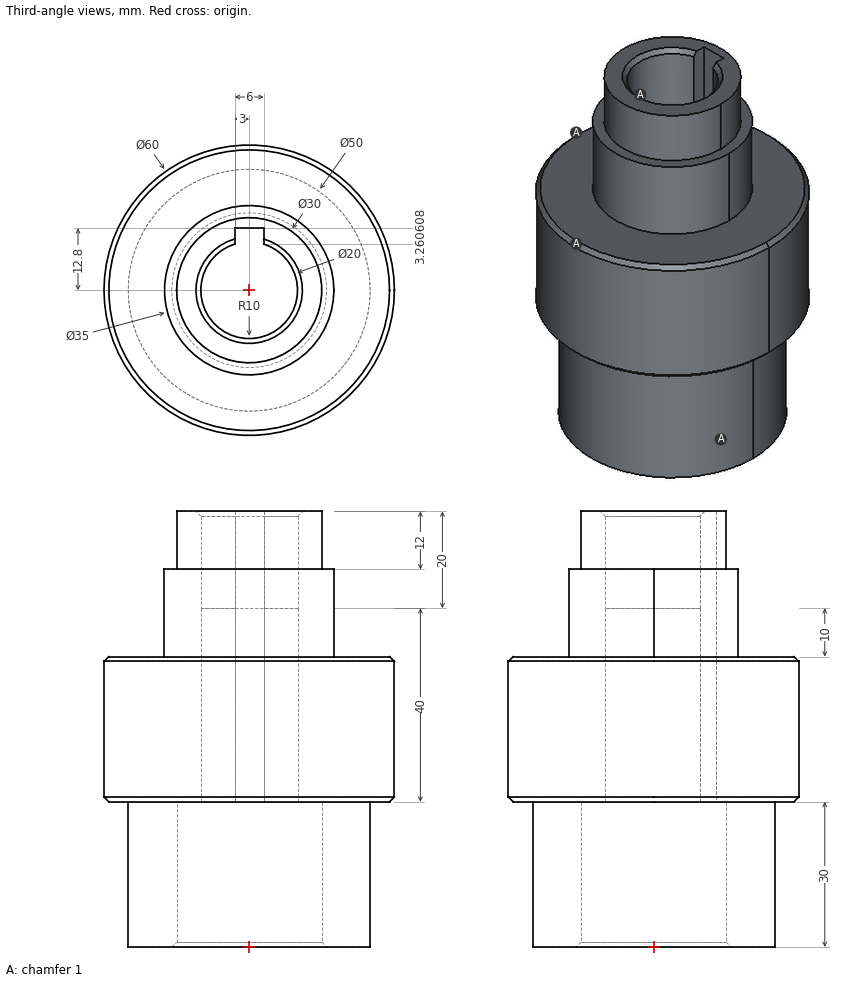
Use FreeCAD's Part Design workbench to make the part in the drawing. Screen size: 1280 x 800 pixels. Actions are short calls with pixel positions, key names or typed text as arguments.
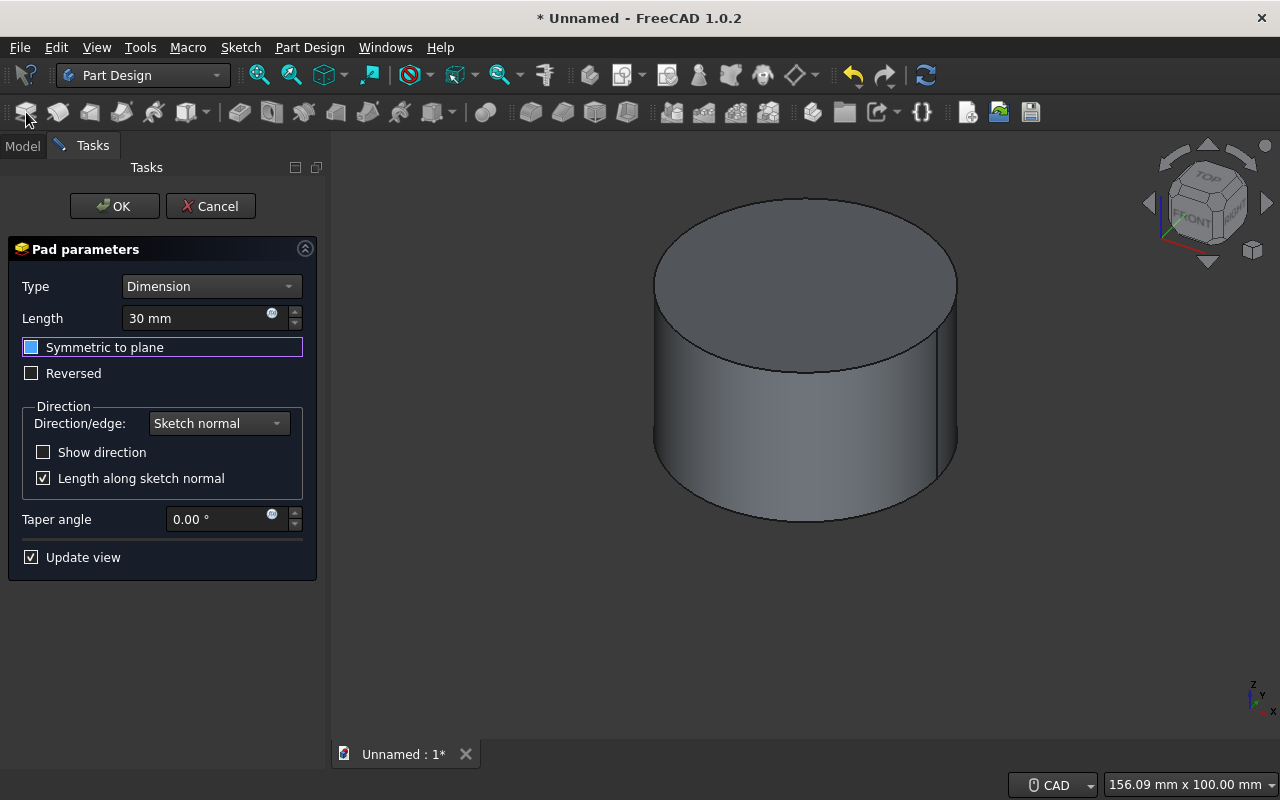
click(115, 206)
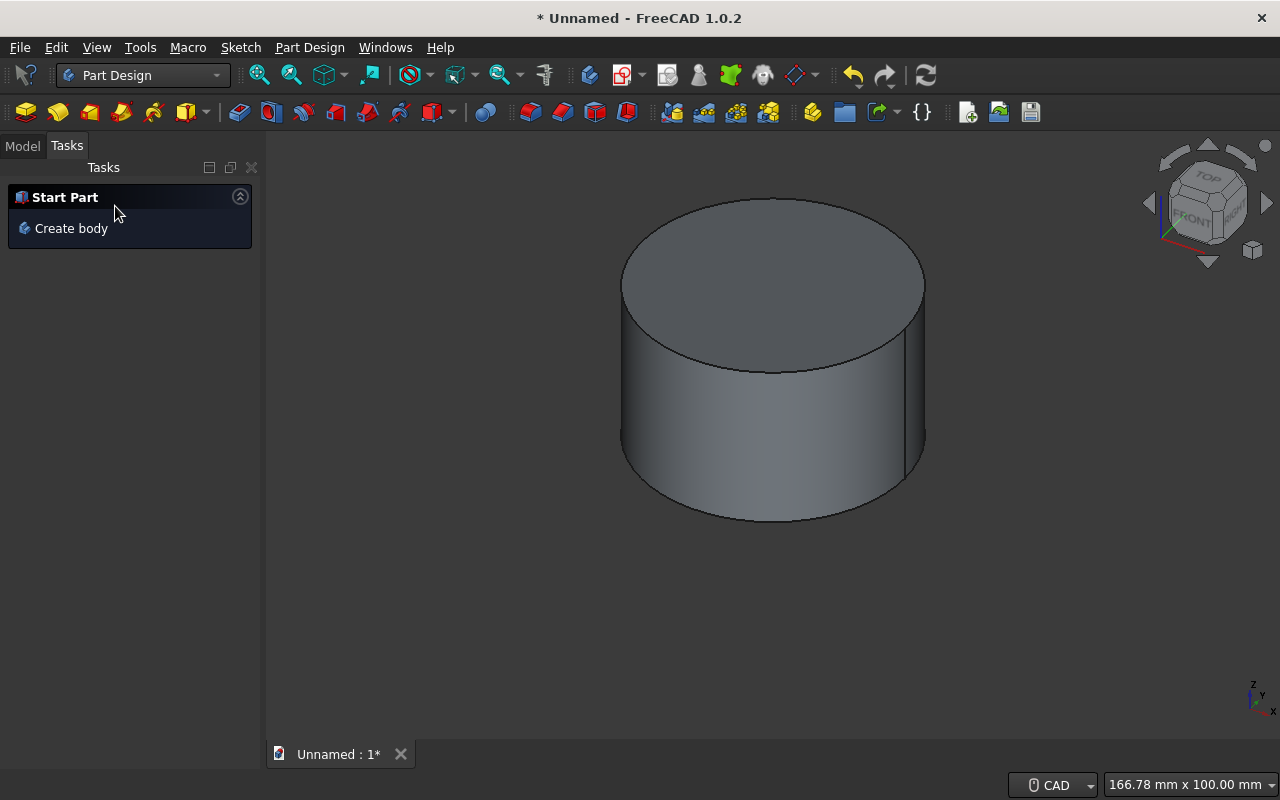
click(773, 285)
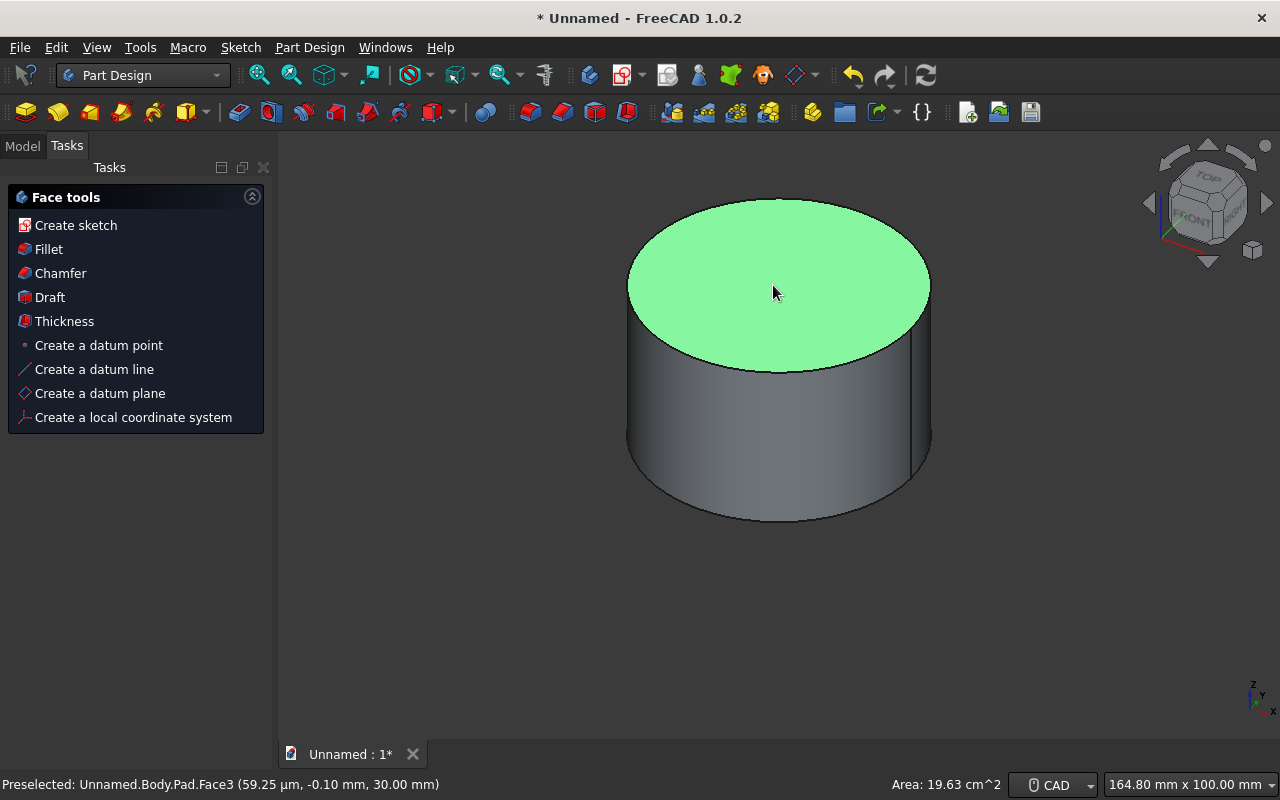
click(622, 76)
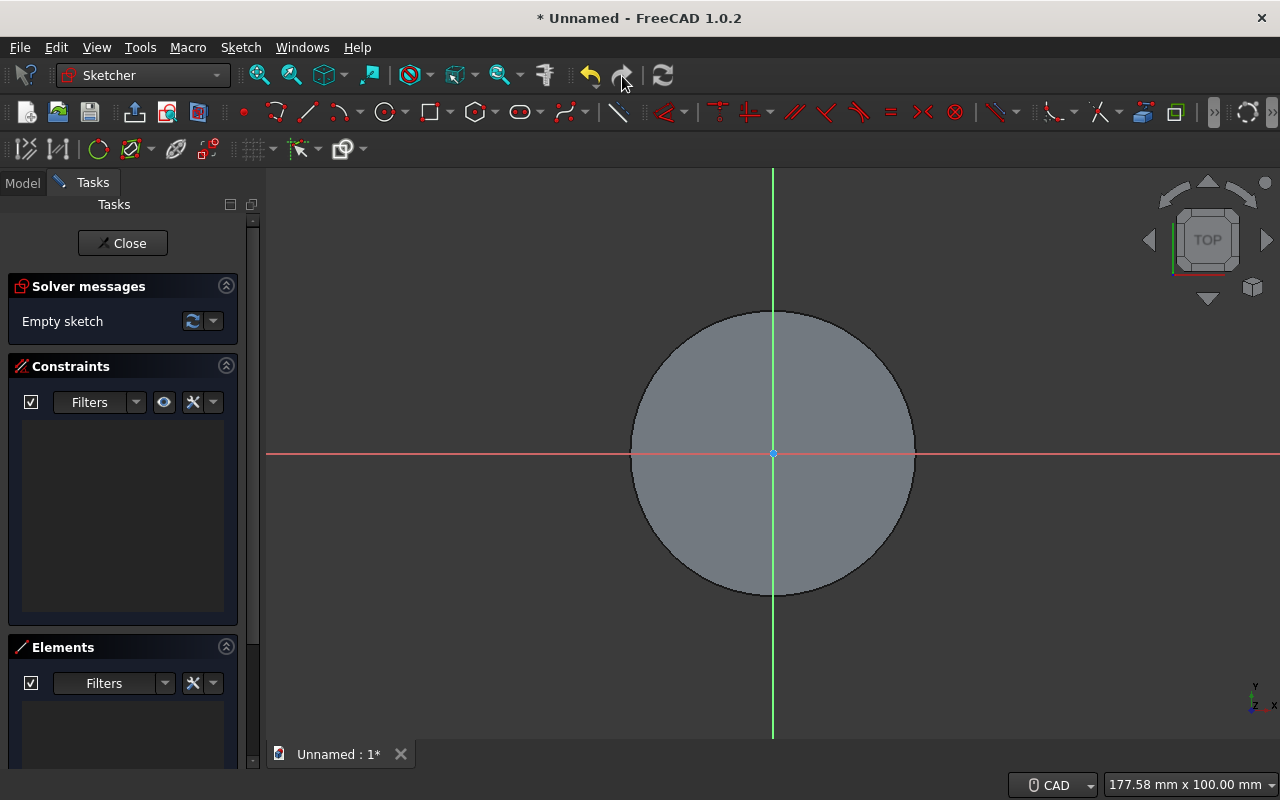
key(g)
key(c)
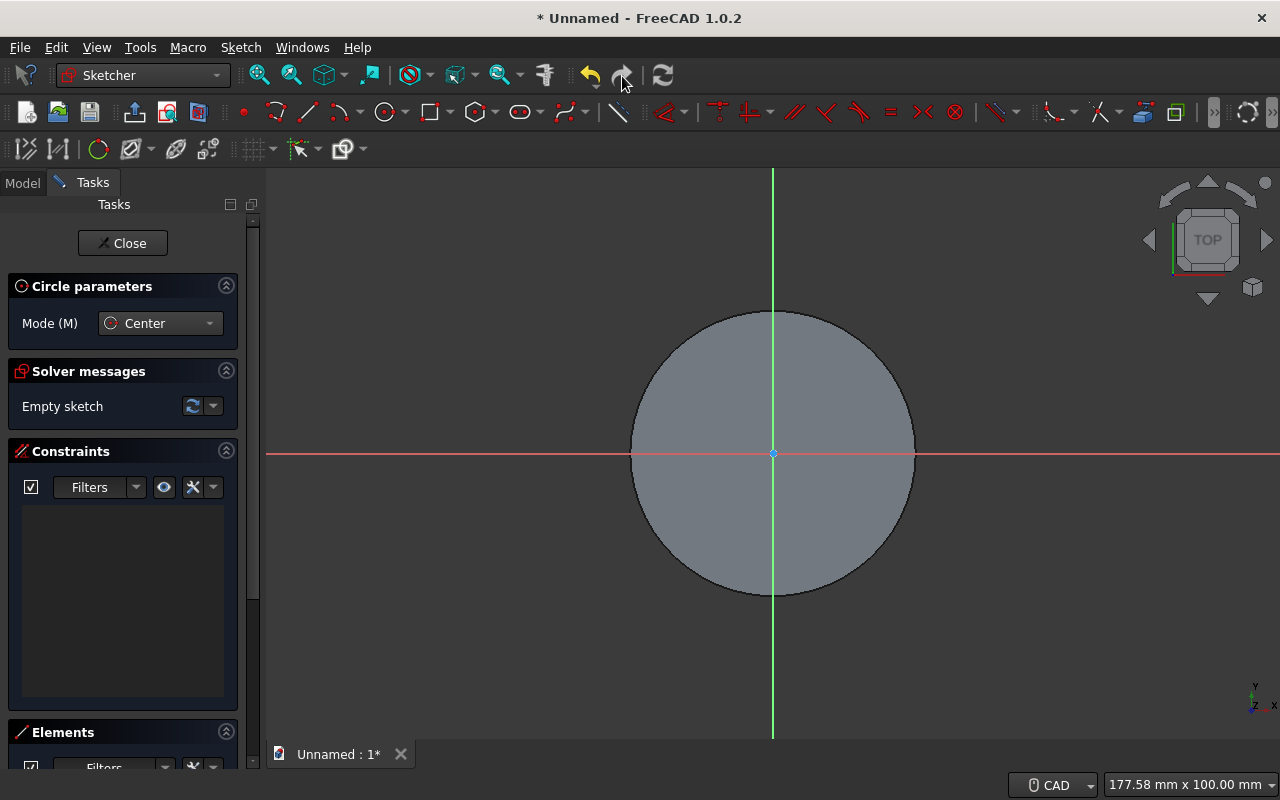
click(773, 454)
move(894, 332)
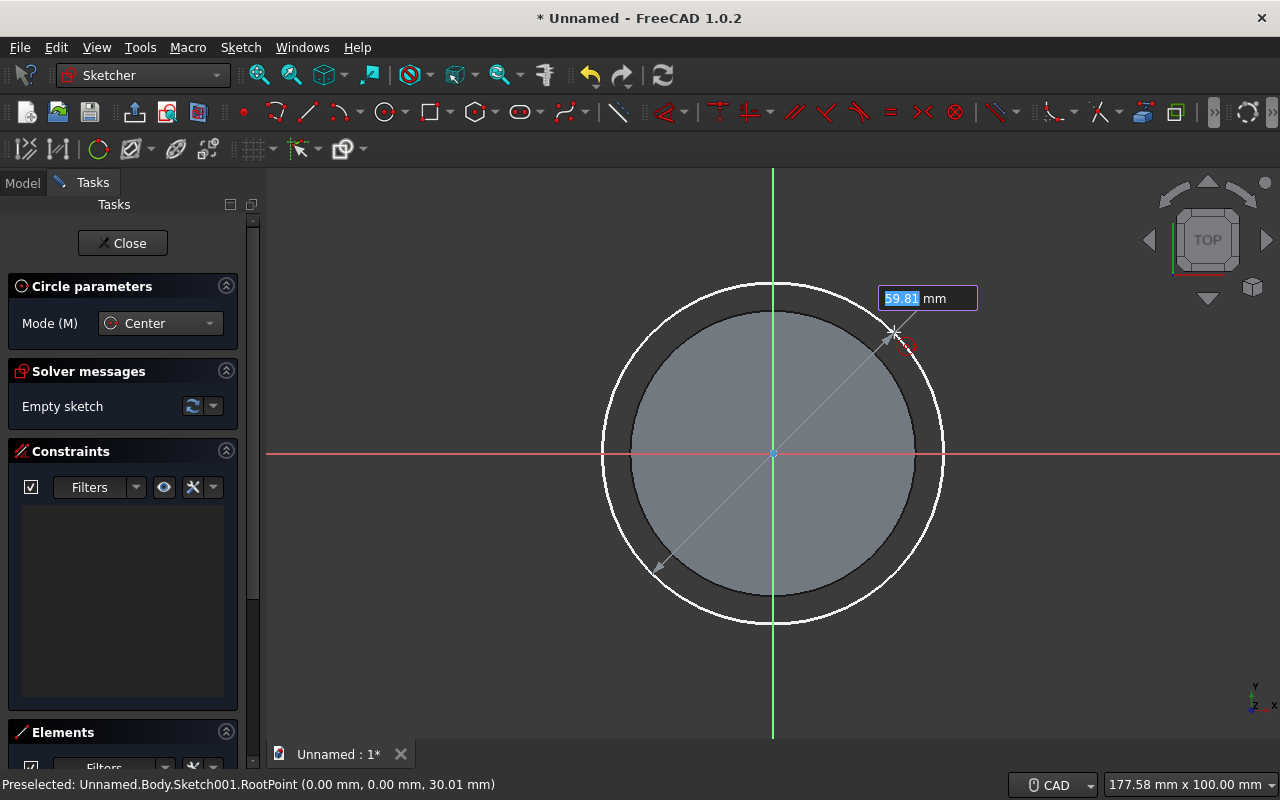
text(60)
key(Return)
key(Escape)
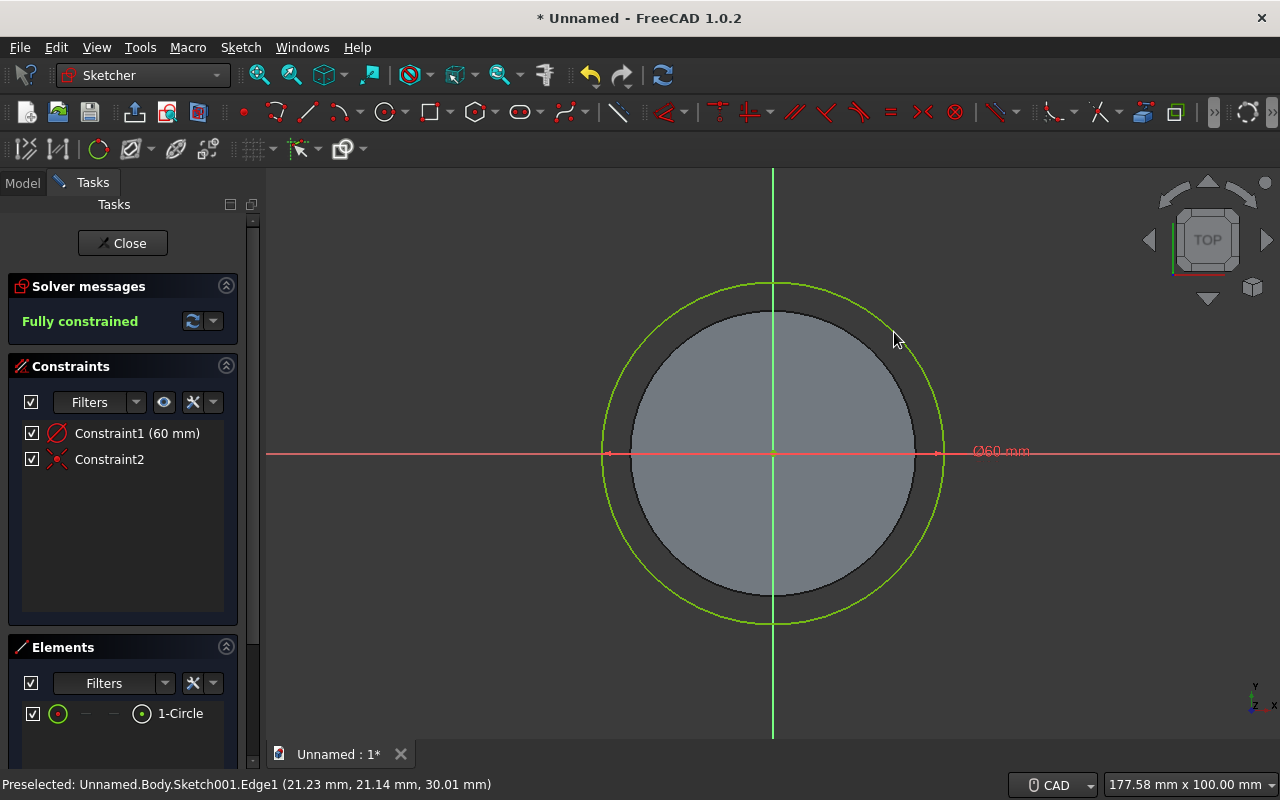
click(123, 243)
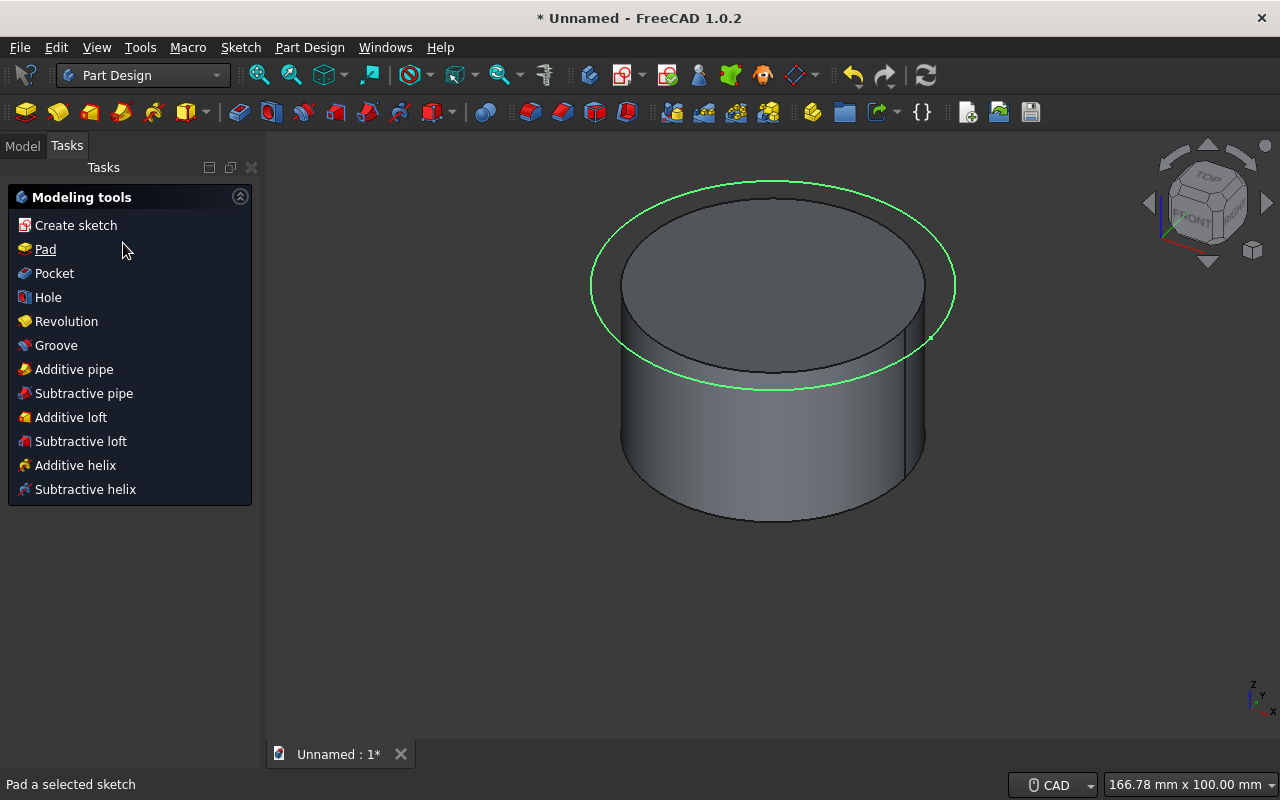
click(26, 112)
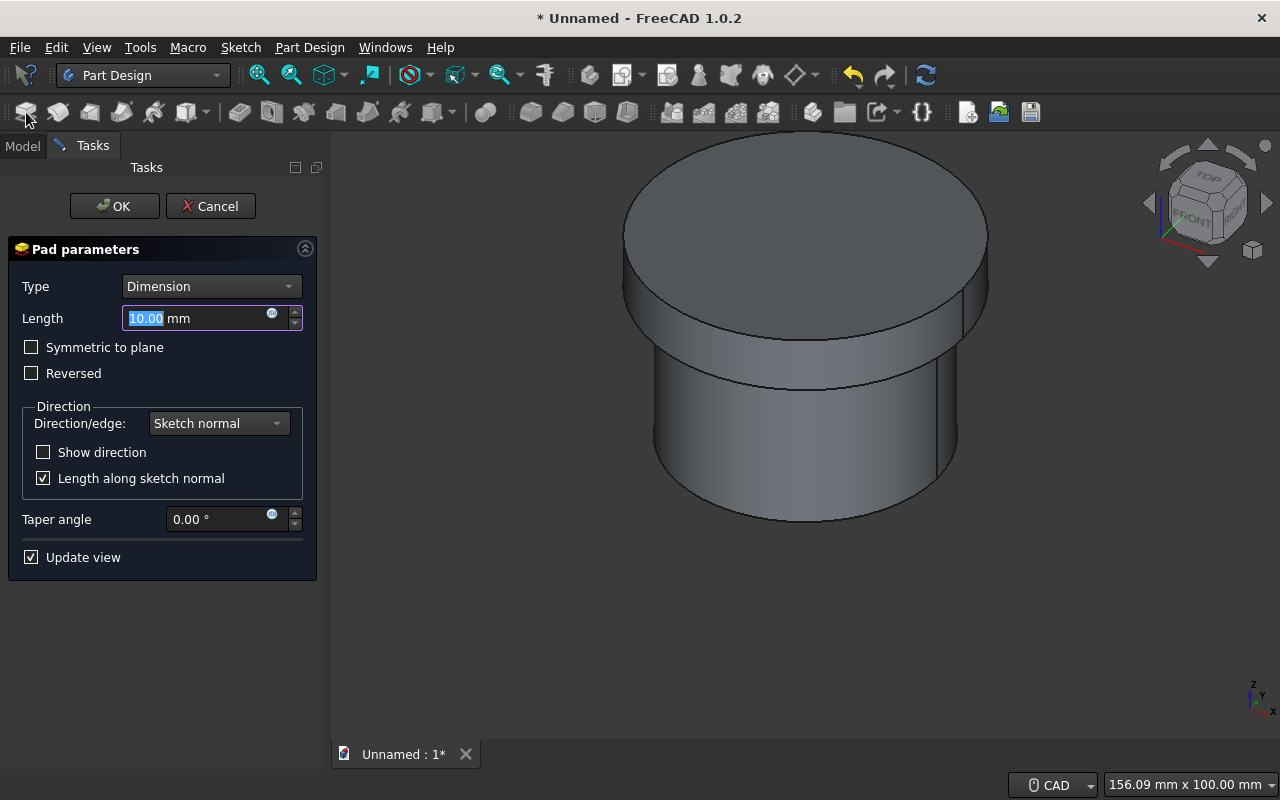
text(40)
key(Tab)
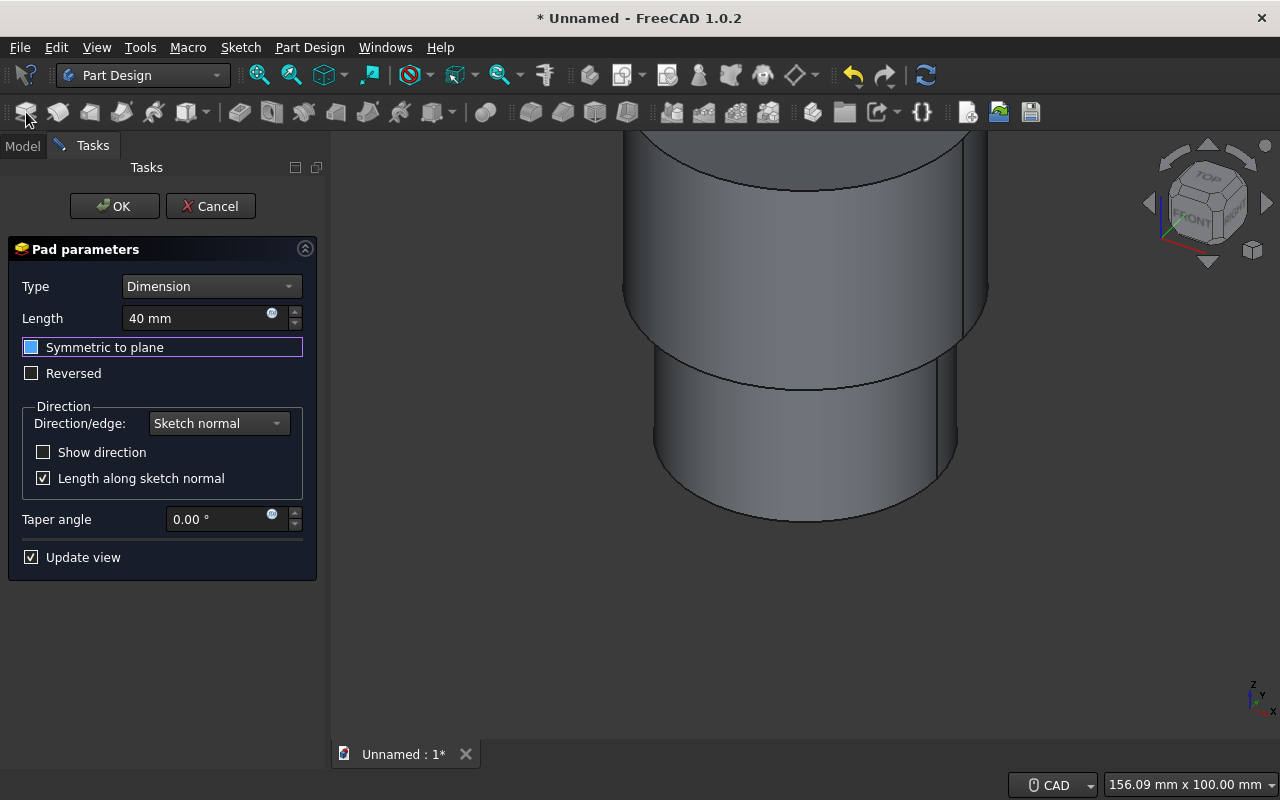
click(115, 206)